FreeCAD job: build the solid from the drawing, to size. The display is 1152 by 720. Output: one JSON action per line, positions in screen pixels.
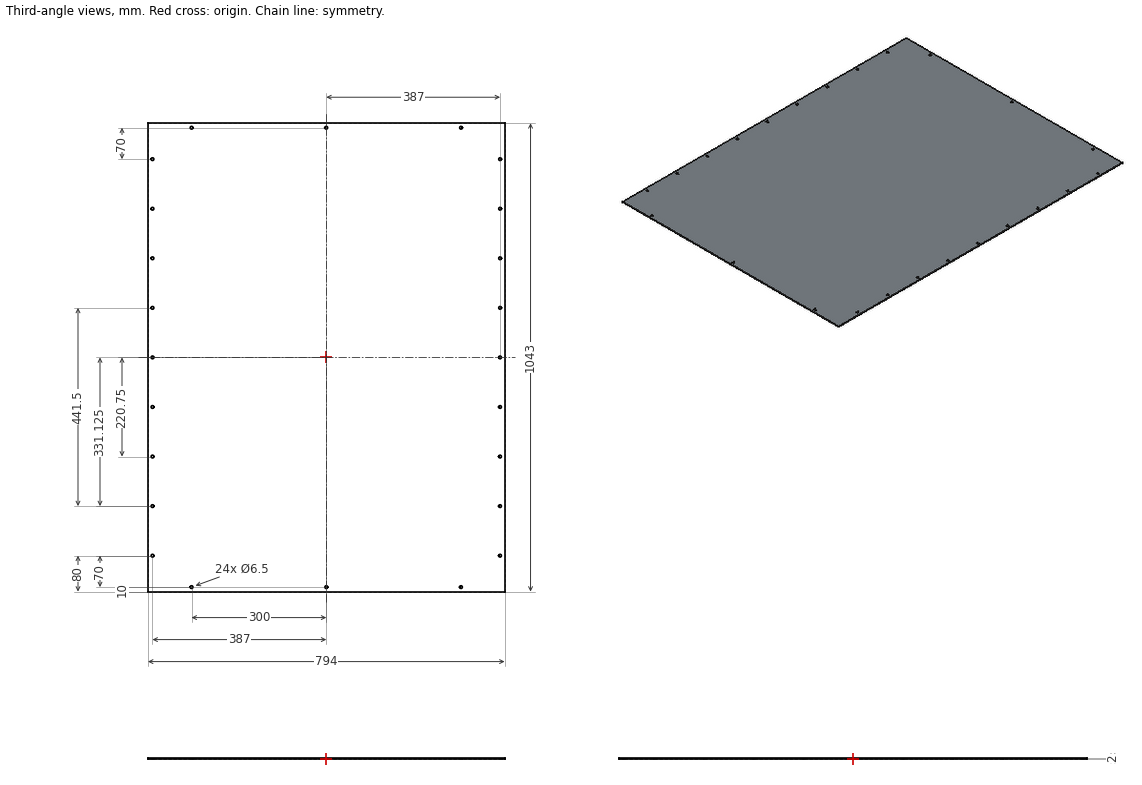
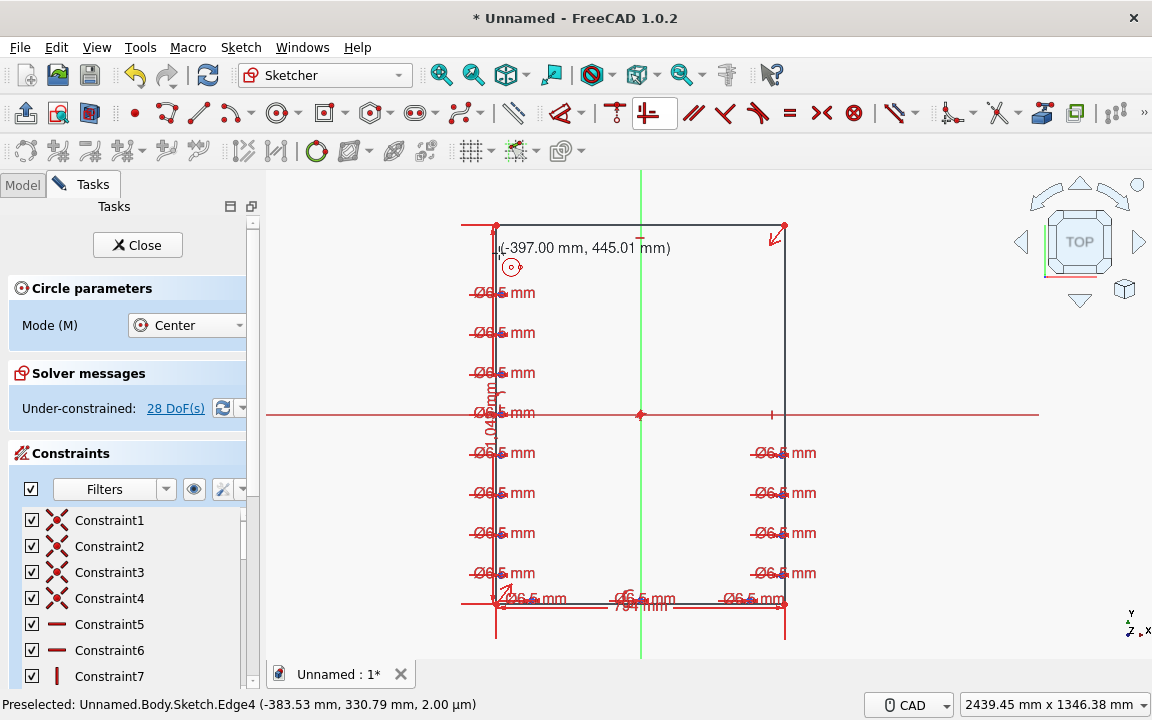
{"action": "scroll", "coordinate": [500, 254], "scroll_direction": "up", "scroll_amount": 8}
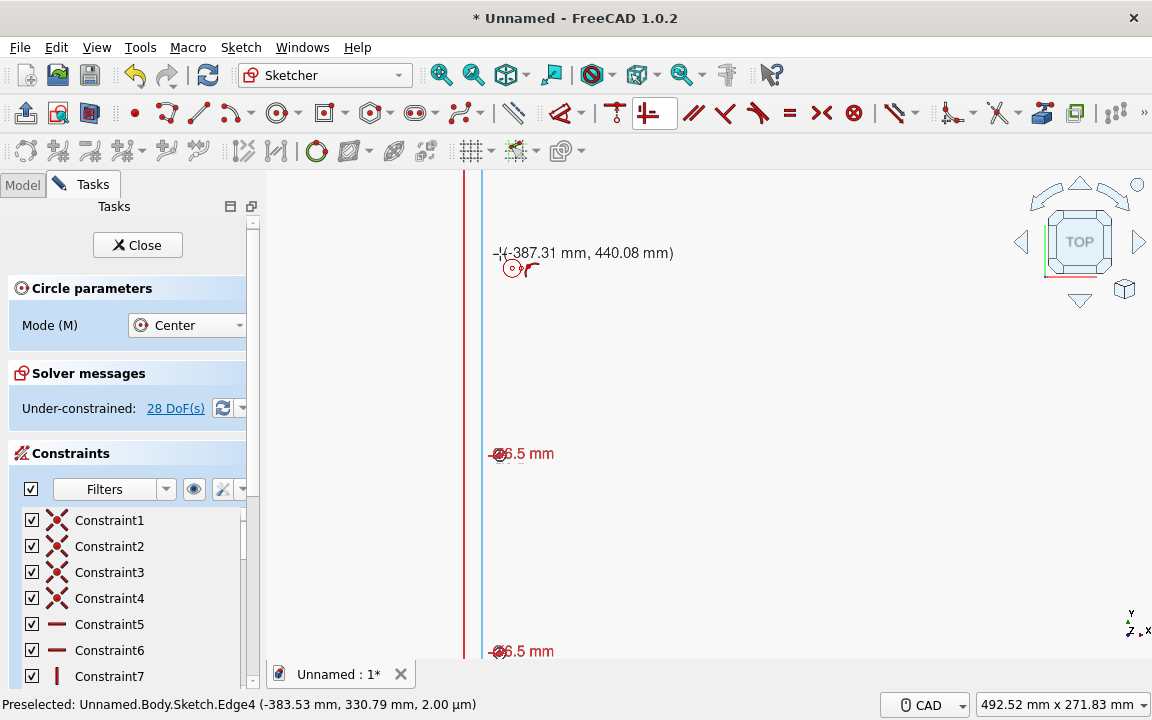
{"action": "left_click", "coordinate": [500, 256]}
{"action": "mouse_move", "coordinate": [504, 252]}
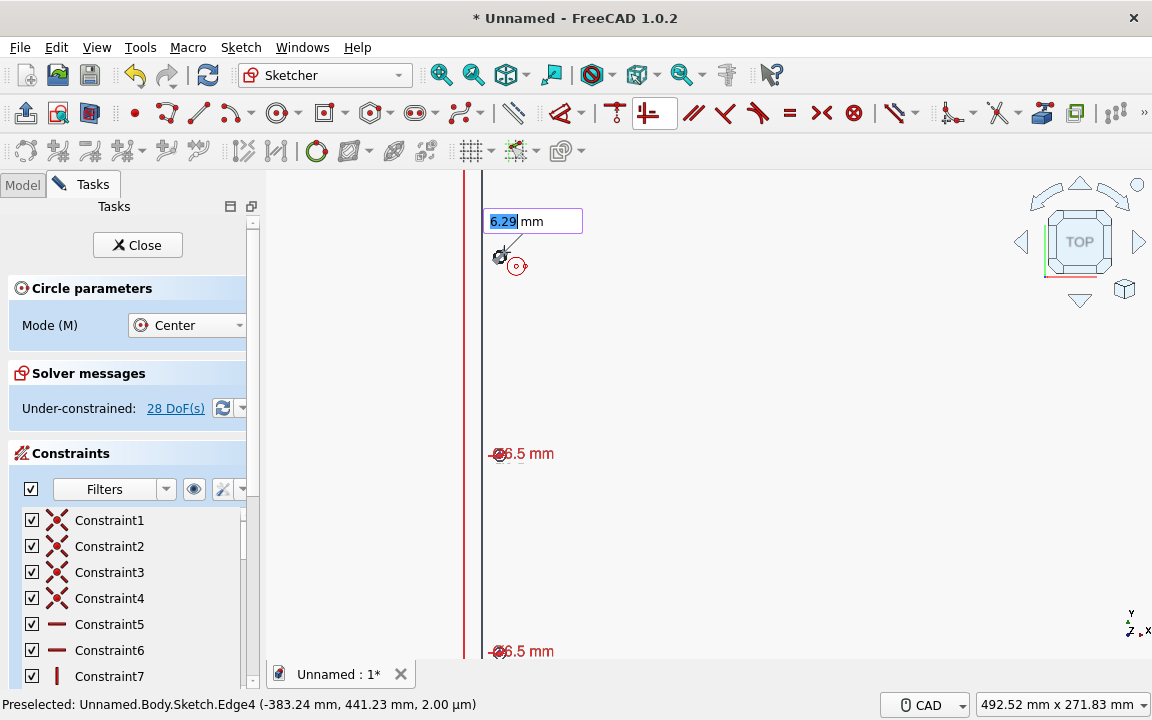
{"action": "type", "text": "6.5"}
{"action": "key", "text": "Return"}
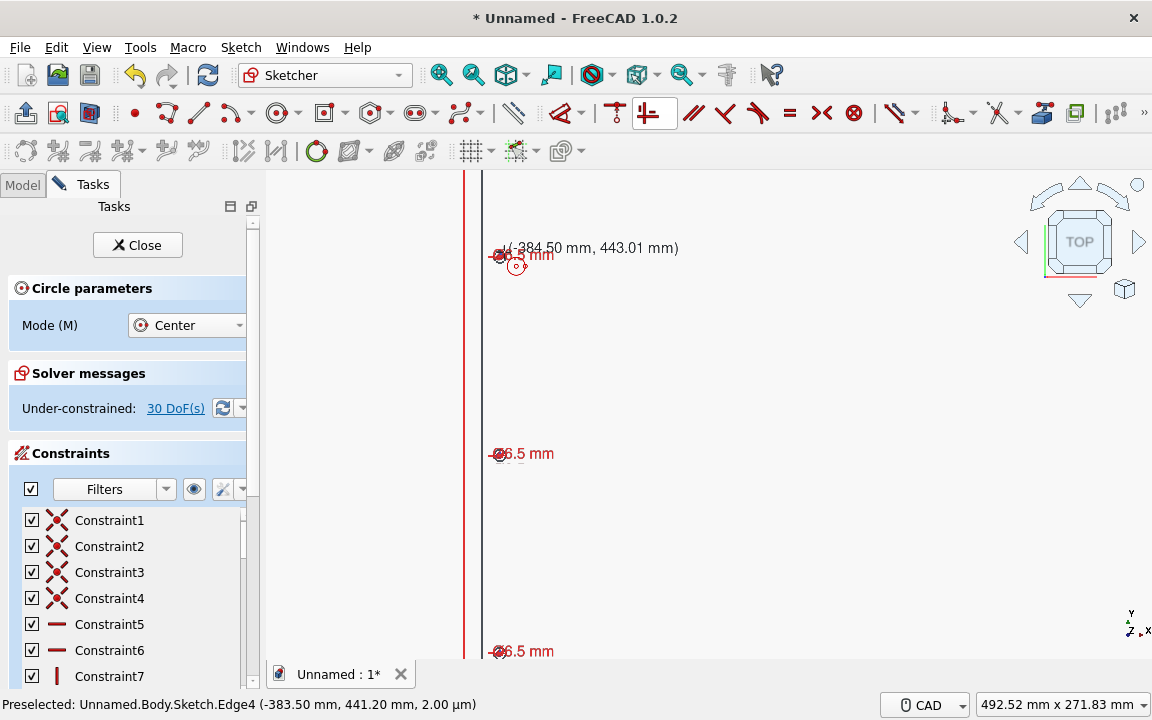
{"action": "scroll", "coordinate": [531, 289], "scroll_direction": "down", "scroll_amount": 9}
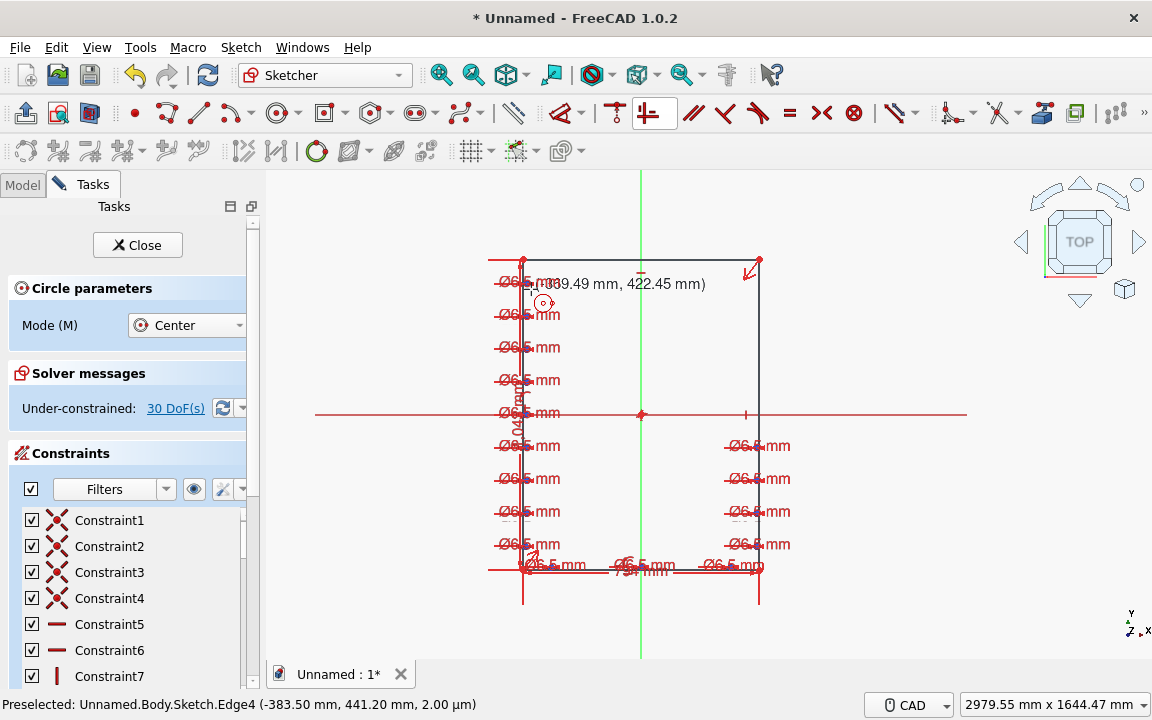
{"action": "scroll", "coordinate": [552, 263], "scroll_direction": "up", "scroll_amount": 16}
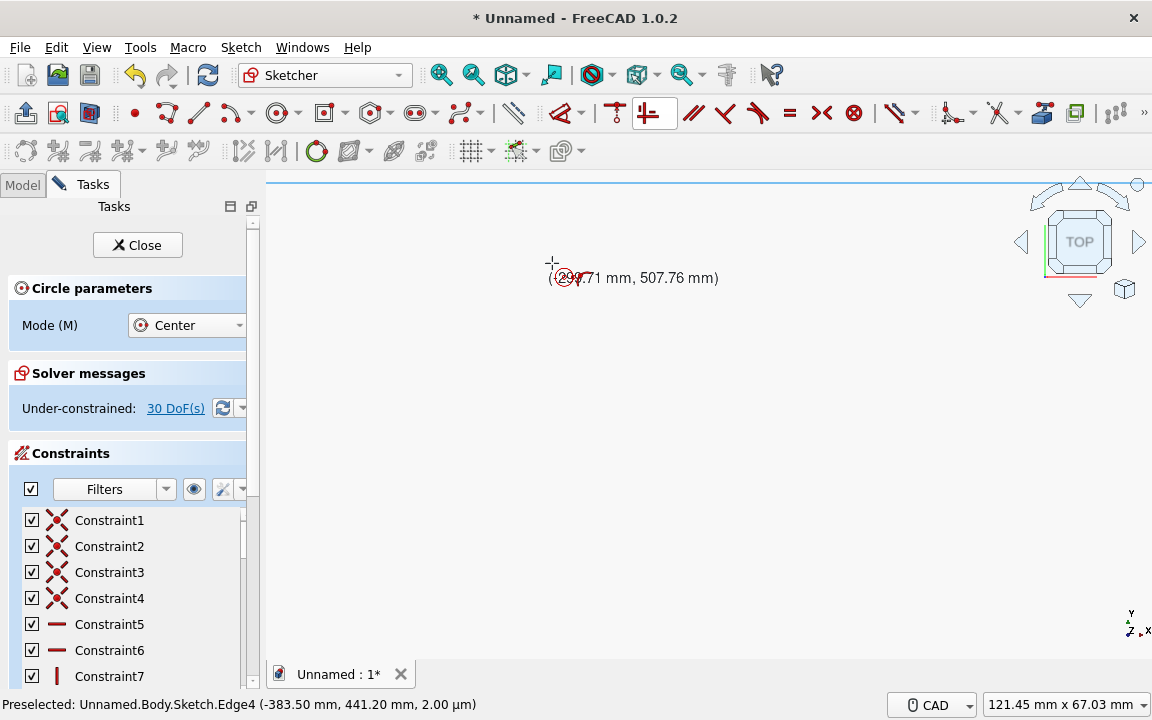
{"action": "scroll", "coordinate": [531, 227], "scroll_direction": "down", "scroll_amount": 15}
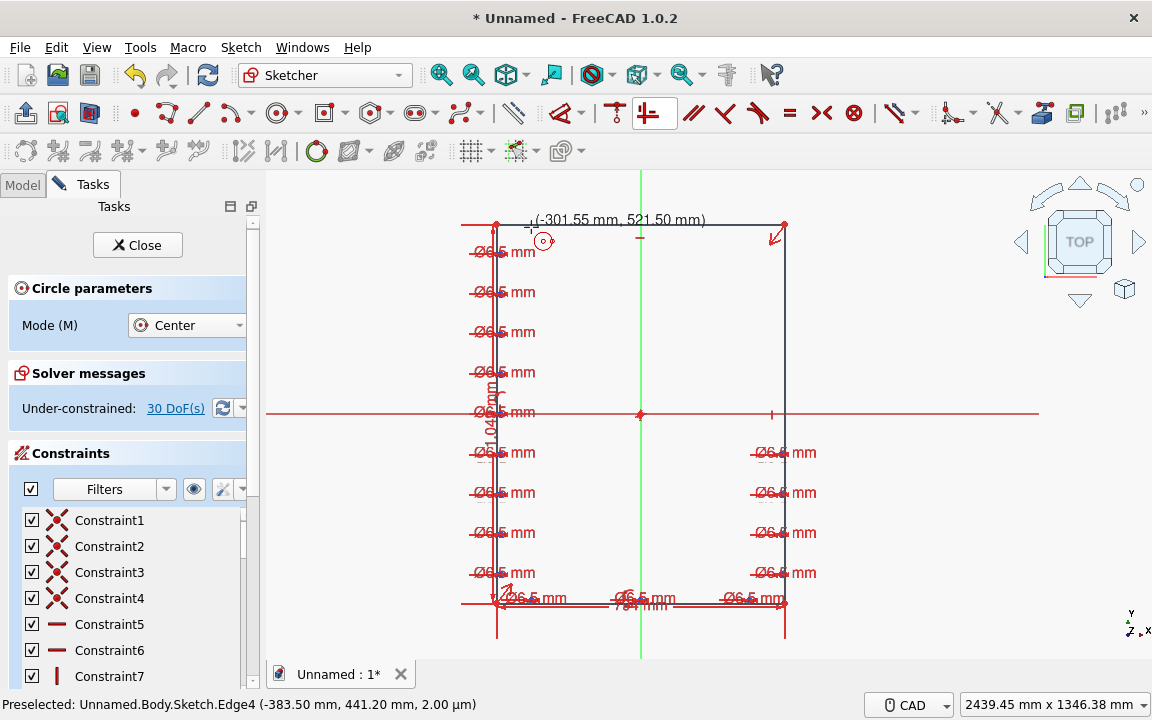
{"action": "scroll", "coordinate": [532, 229], "scroll_direction": "up", "scroll_amount": 8}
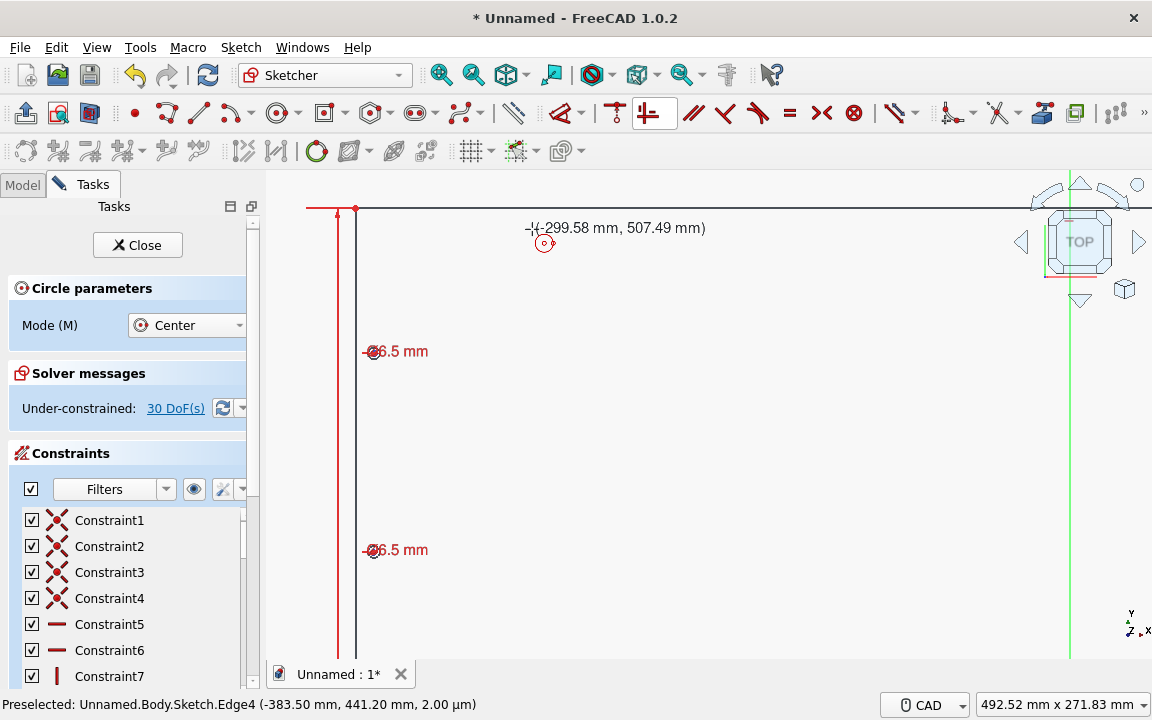
{"action": "left_click", "coordinate": [530, 226]}
{"action": "mouse_move", "coordinate": [534, 230]}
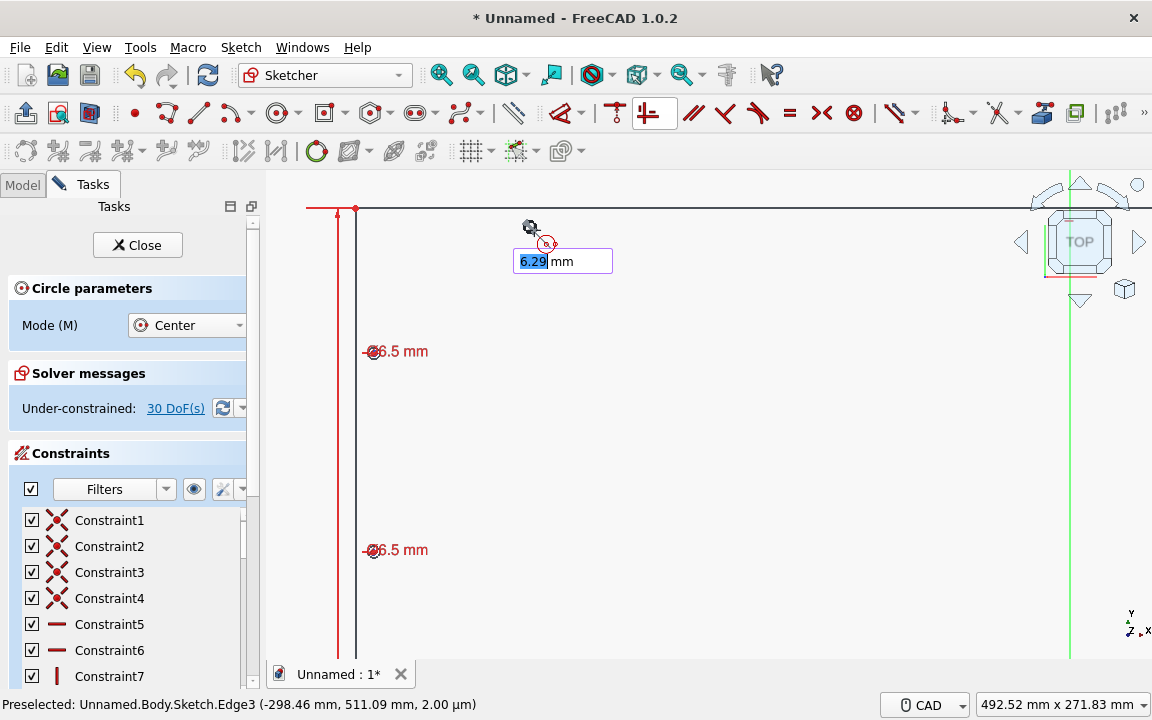
{"action": "type", "text": "6.5"}
{"action": "key", "text": "Return"}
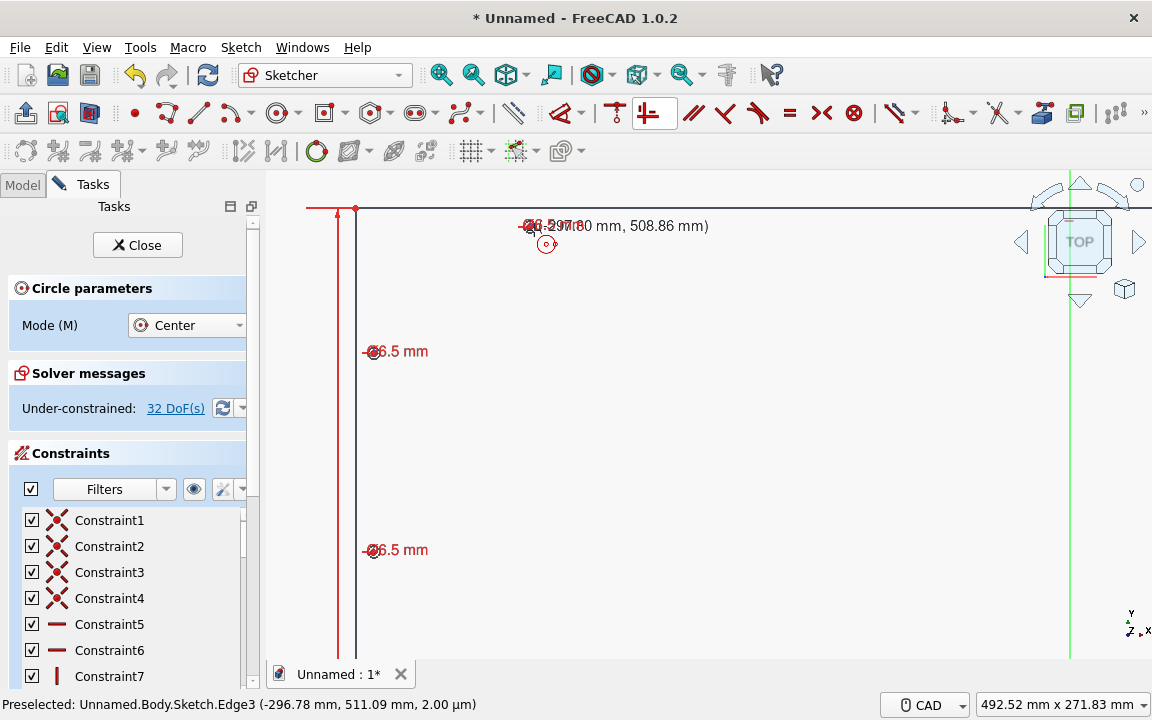
{"action": "scroll", "coordinate": [555, 270], "scroll_direction": "down", "scroll_amount": 9}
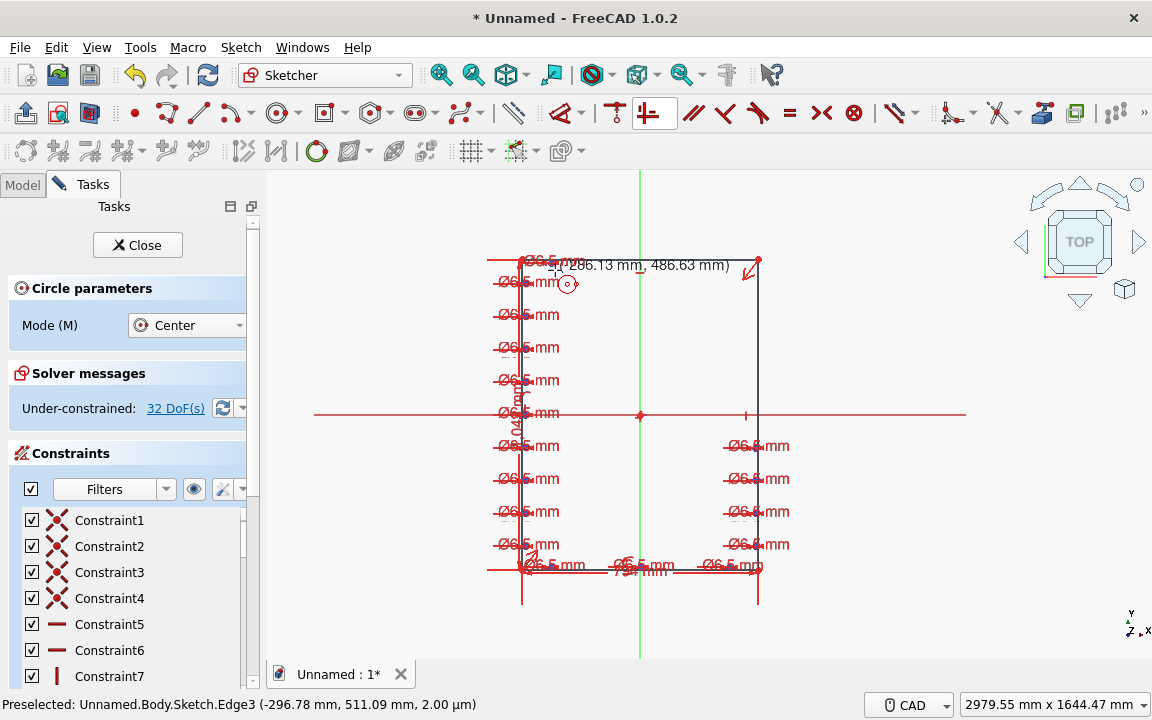
{"action": "scroll", "coordinate": [640, 263], "scroll_direction": "up", "scroll_amount": 16}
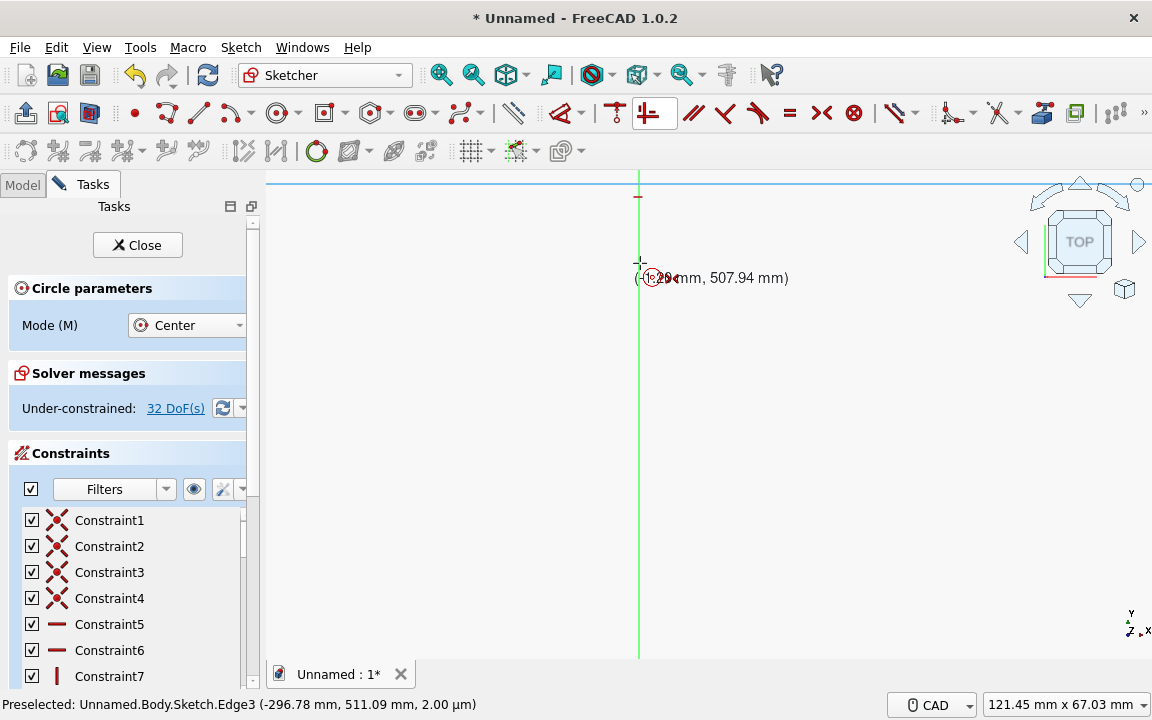
{"action": "scroll", "coordinate": [641, 227], "scroll_direction": "down", "scroll_amount": 15}